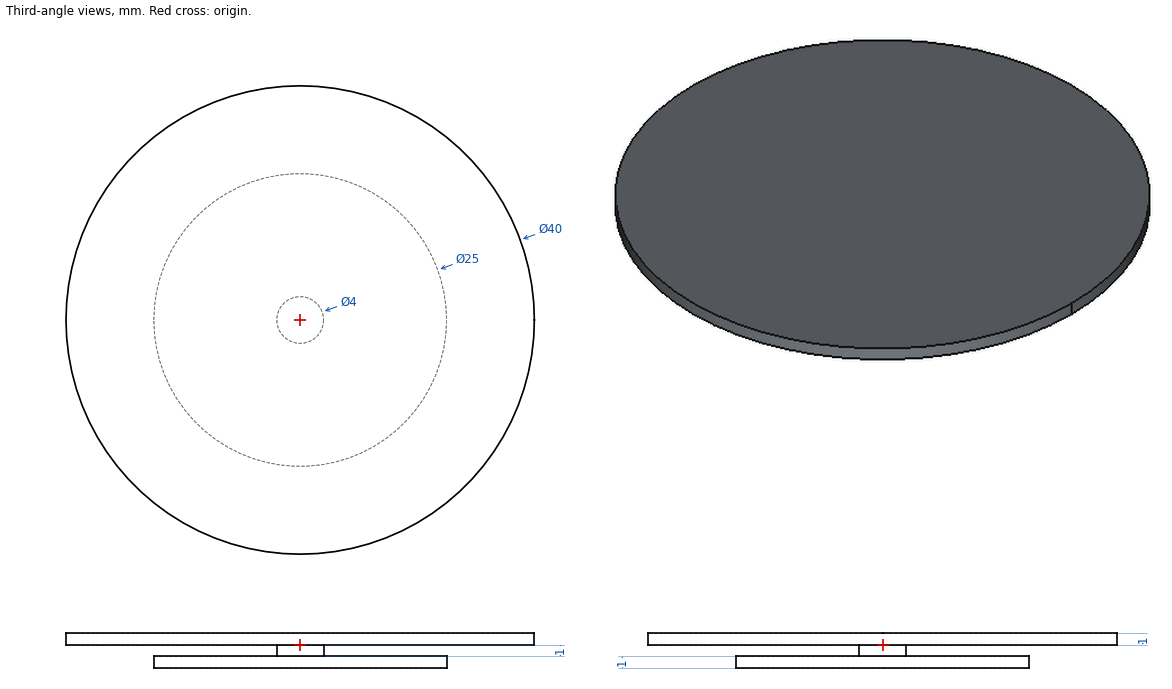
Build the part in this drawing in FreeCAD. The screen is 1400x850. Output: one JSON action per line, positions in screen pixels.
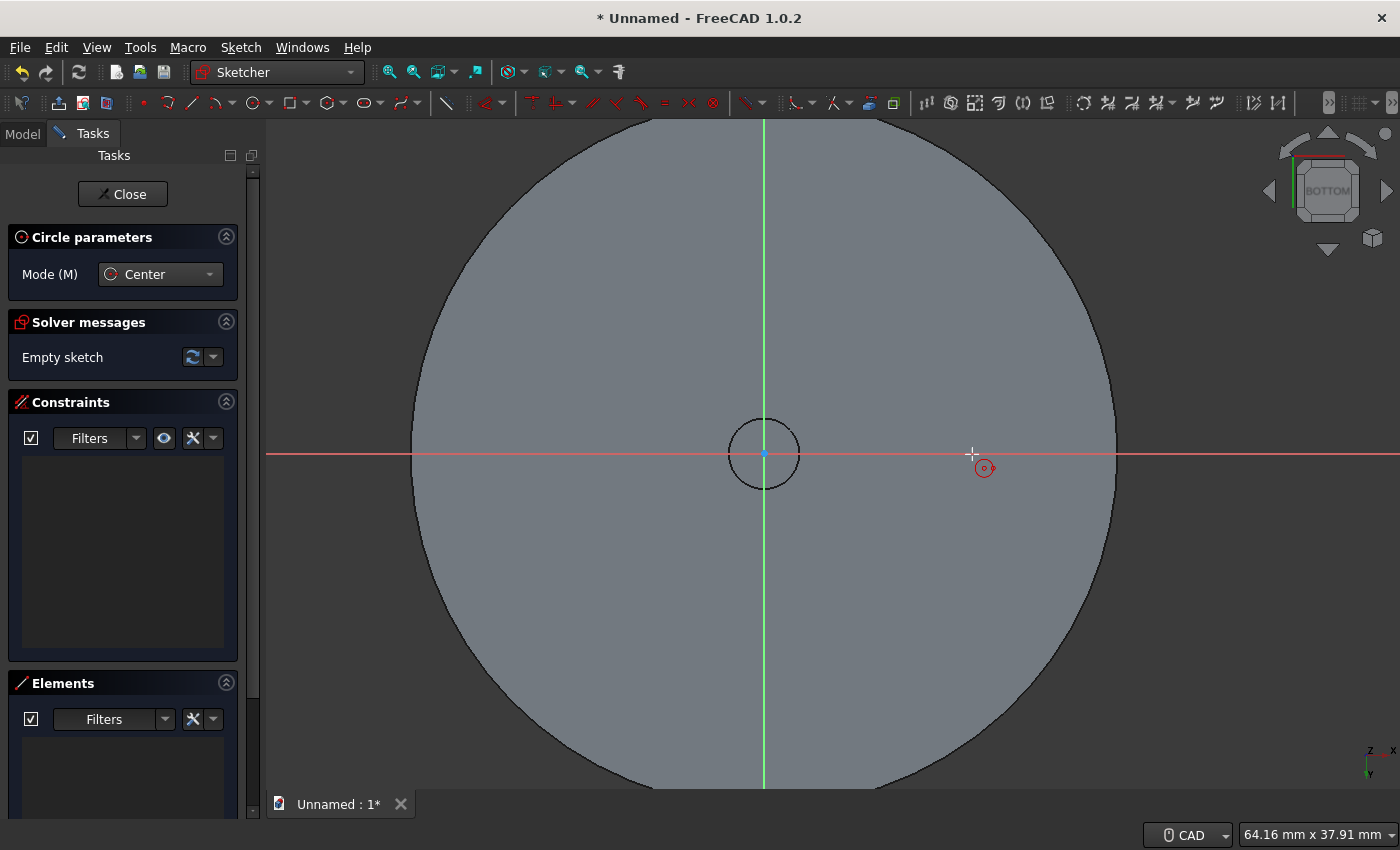
{"action": "left_click", "coordinate": [764, 454]}
{"action": "left_click", "coordinate": [920, 298]}
{"action": "key", "text": "Escape"}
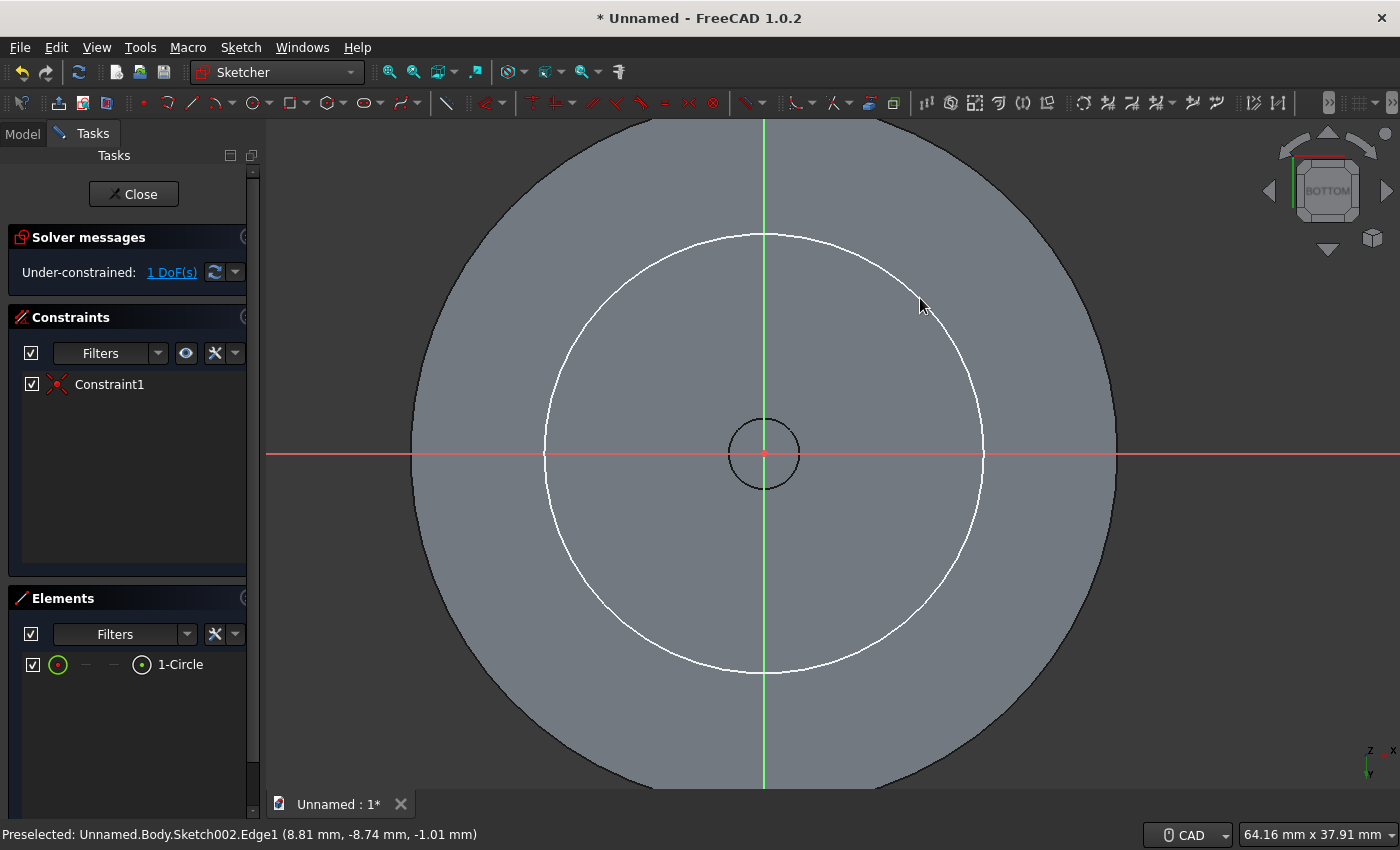
{"action": "key", "text": "d"}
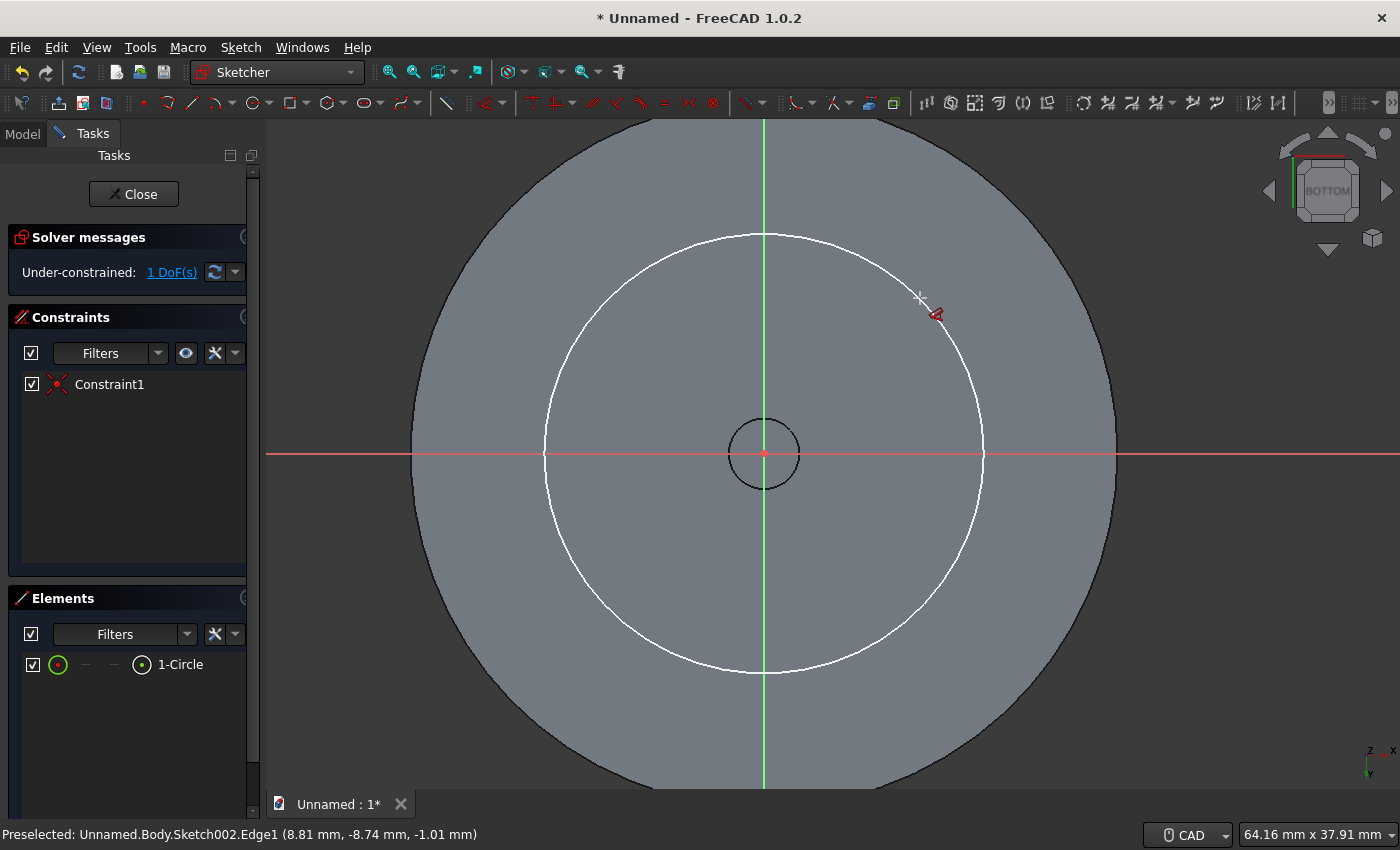
{"action": "left_click", "coordinate": [919, 298]}
{"action": "left_click", "coordinate": [942, 275]}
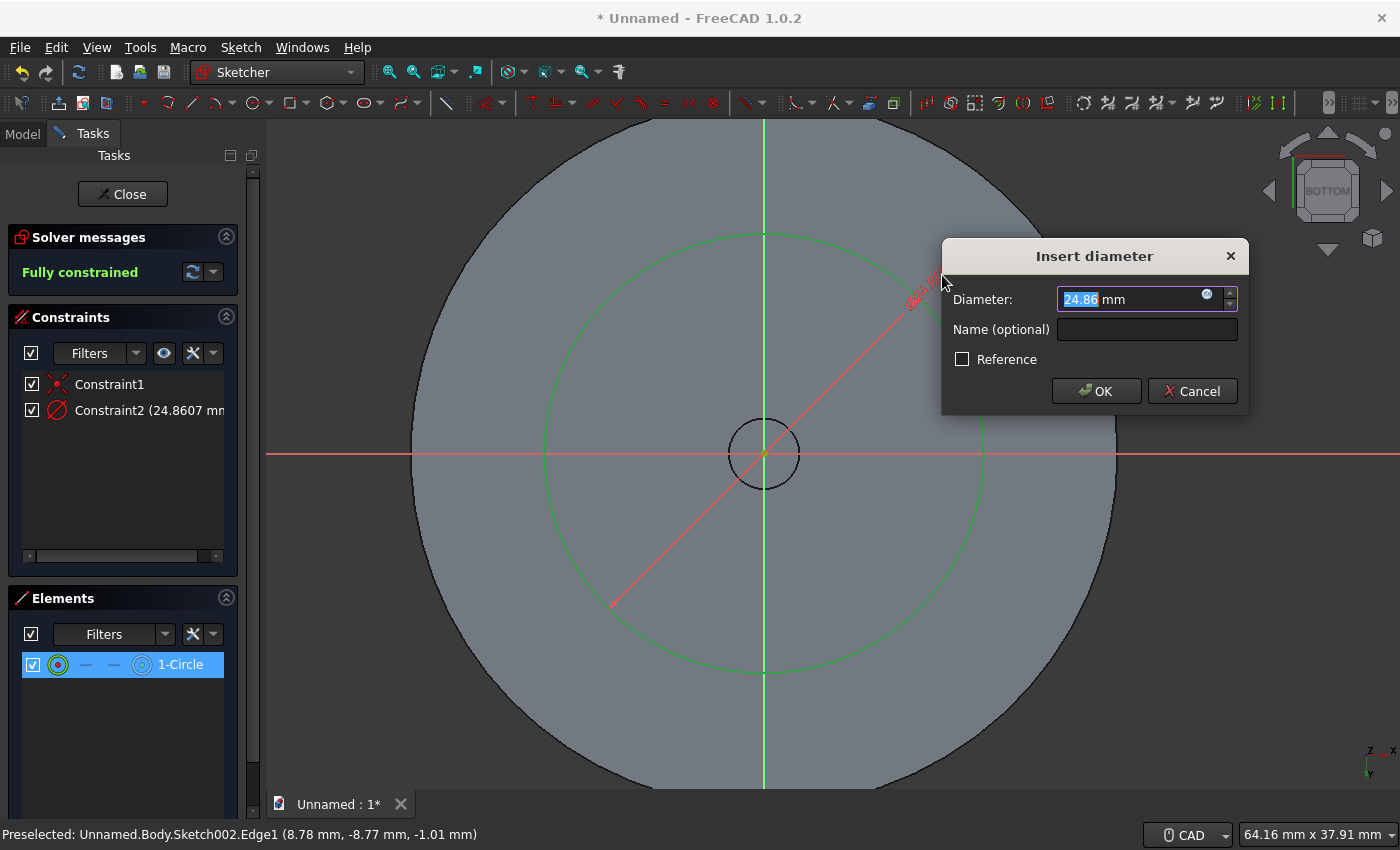
{"action": "type", "text": "25"}
{"action": "key", "text": "Return"}
{"action": "key", "text": "Escape"}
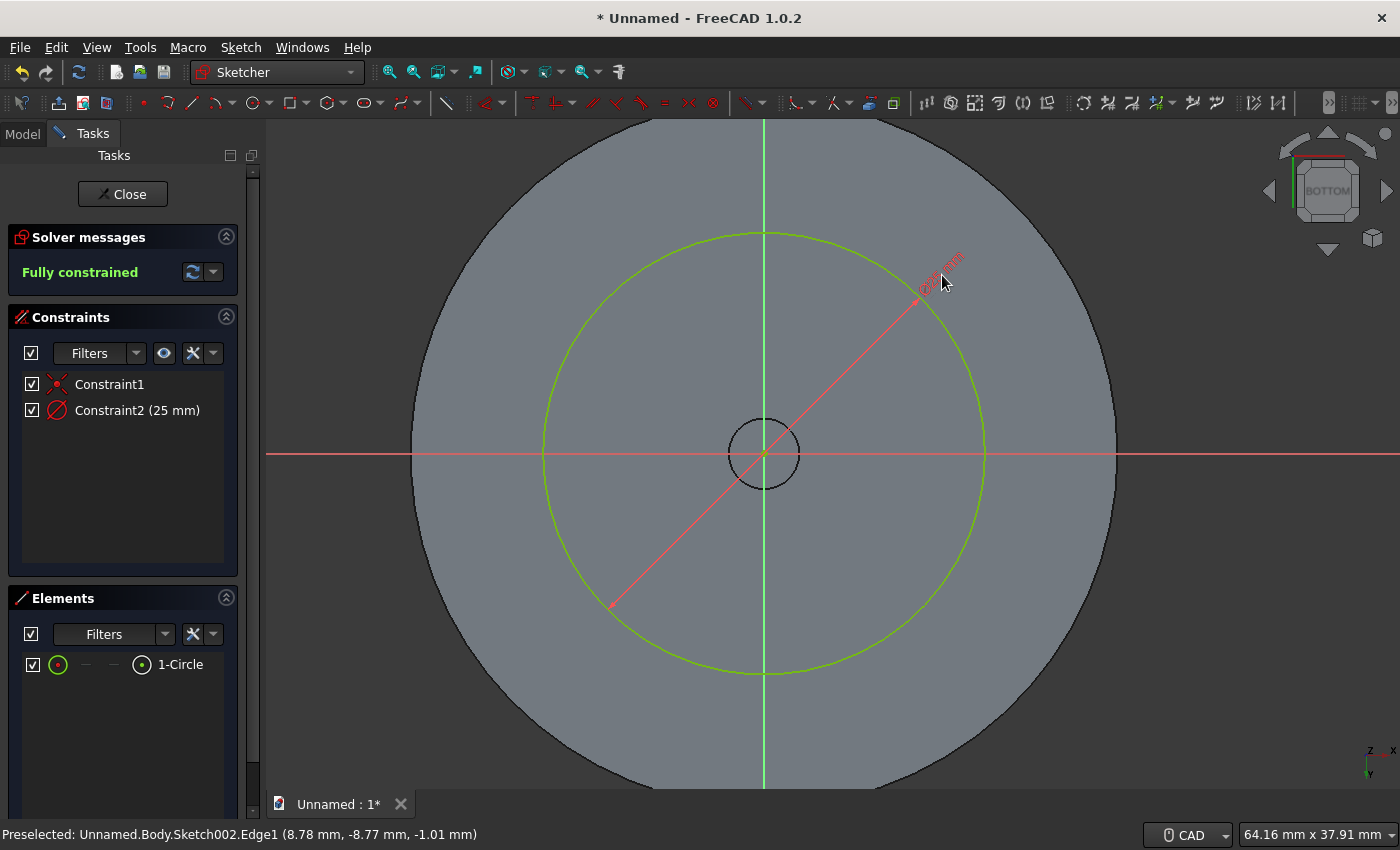
{"action": "left_click", "coordinate": [123, 194]}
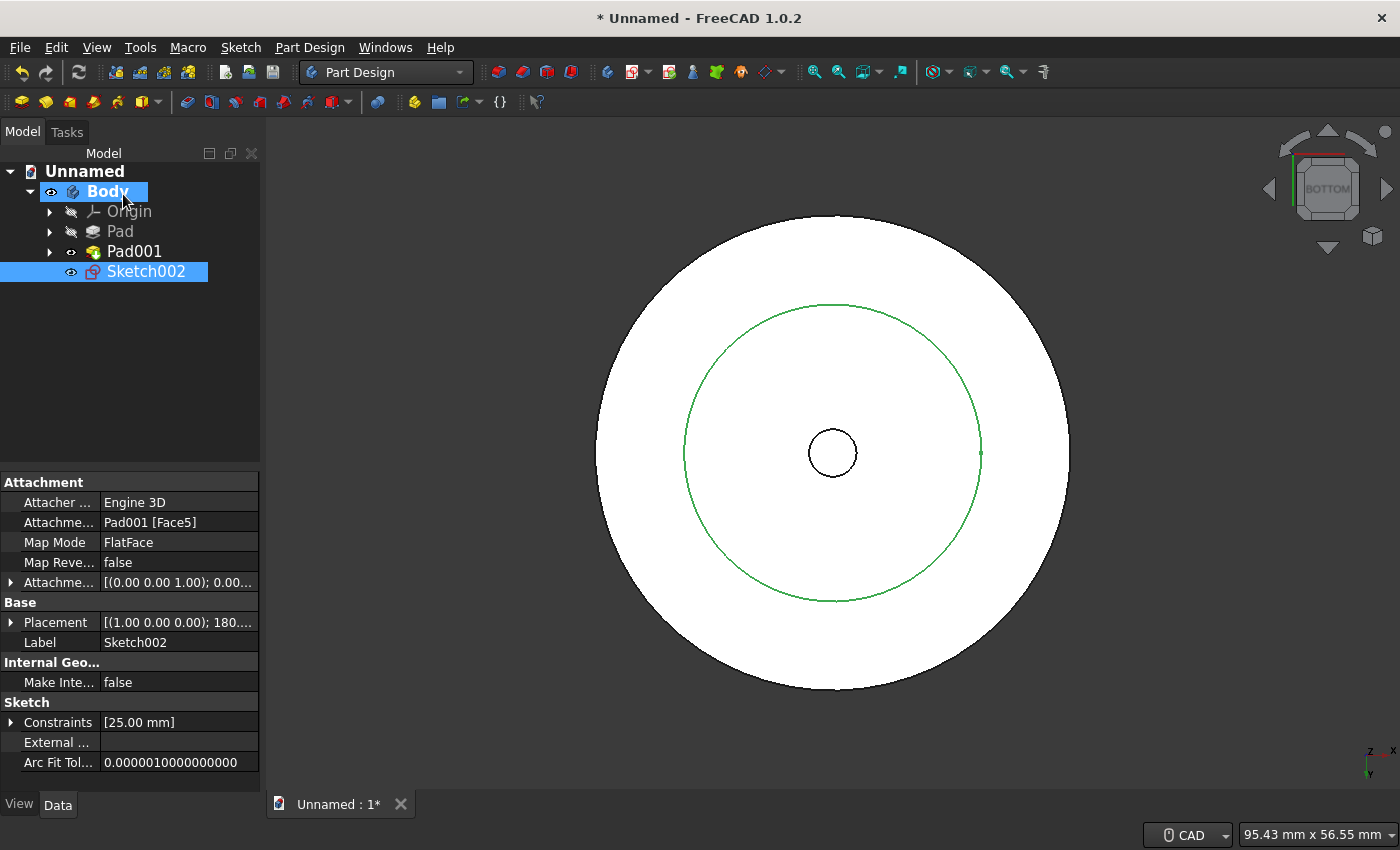
{"action": "left_click", "coordinate": [22, 102]}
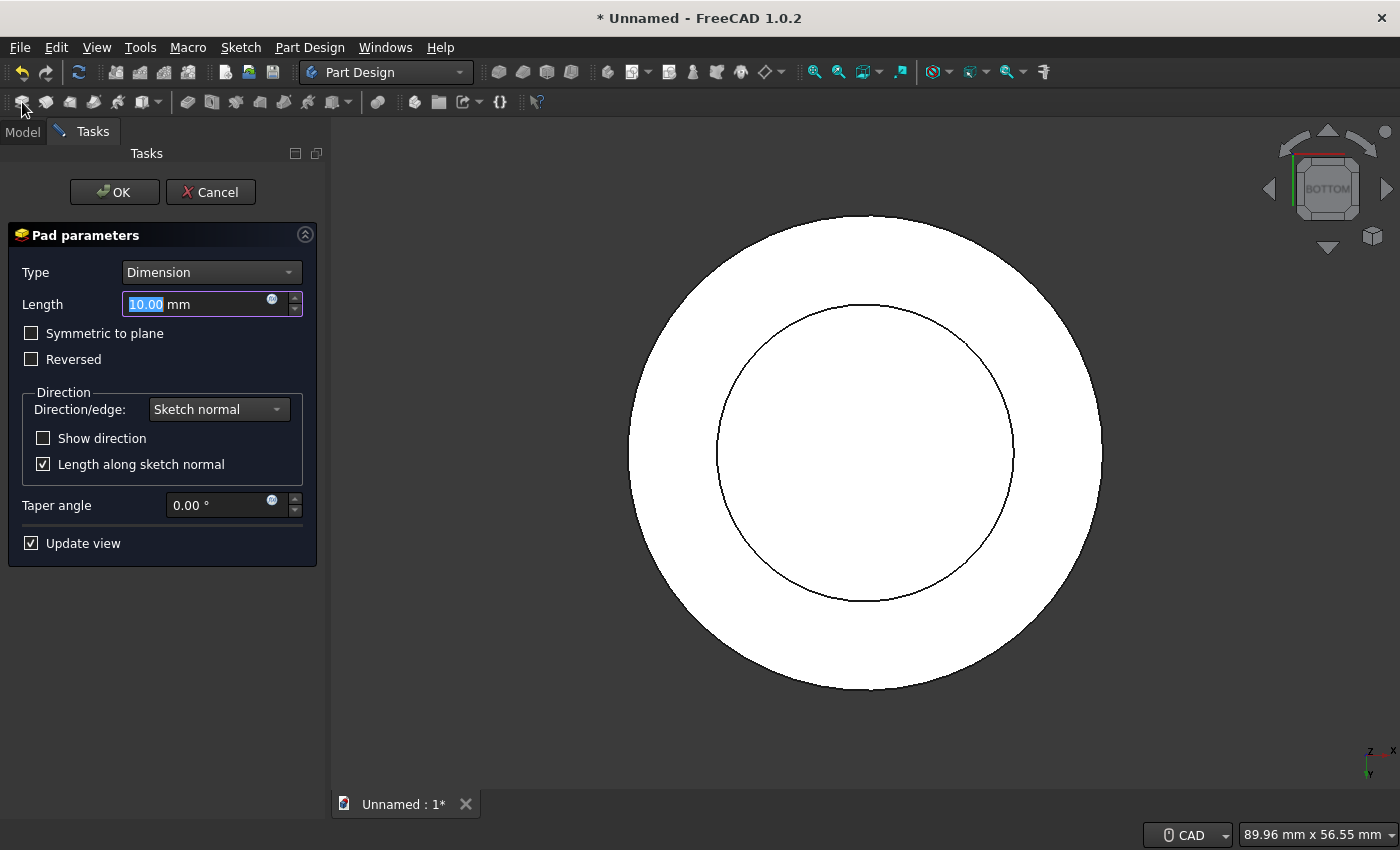
{"action": "type", "text": "1"}
{"action": "key", "text": "Tab"}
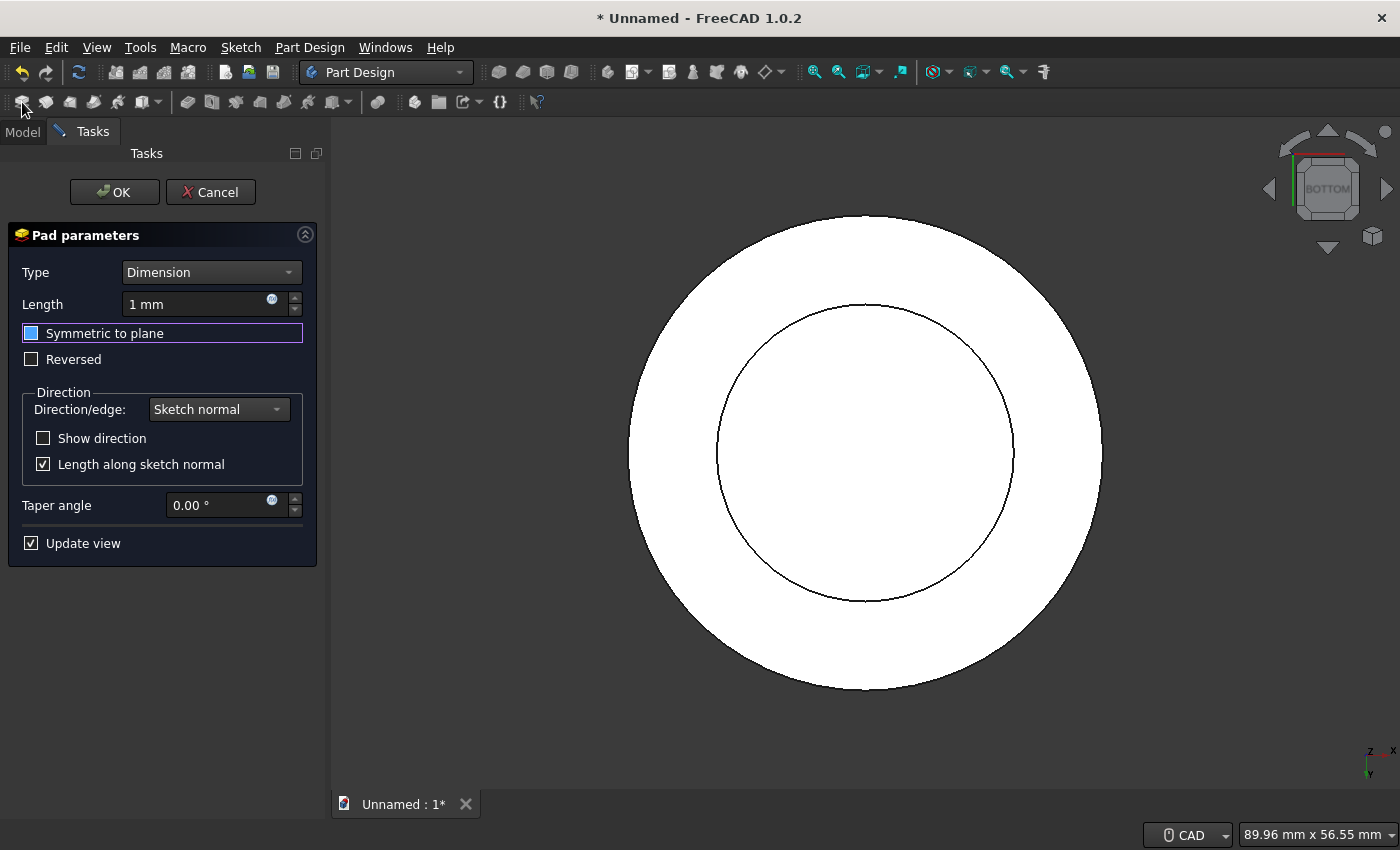
{"action": "left_click", "coordinate": [115, 192]}